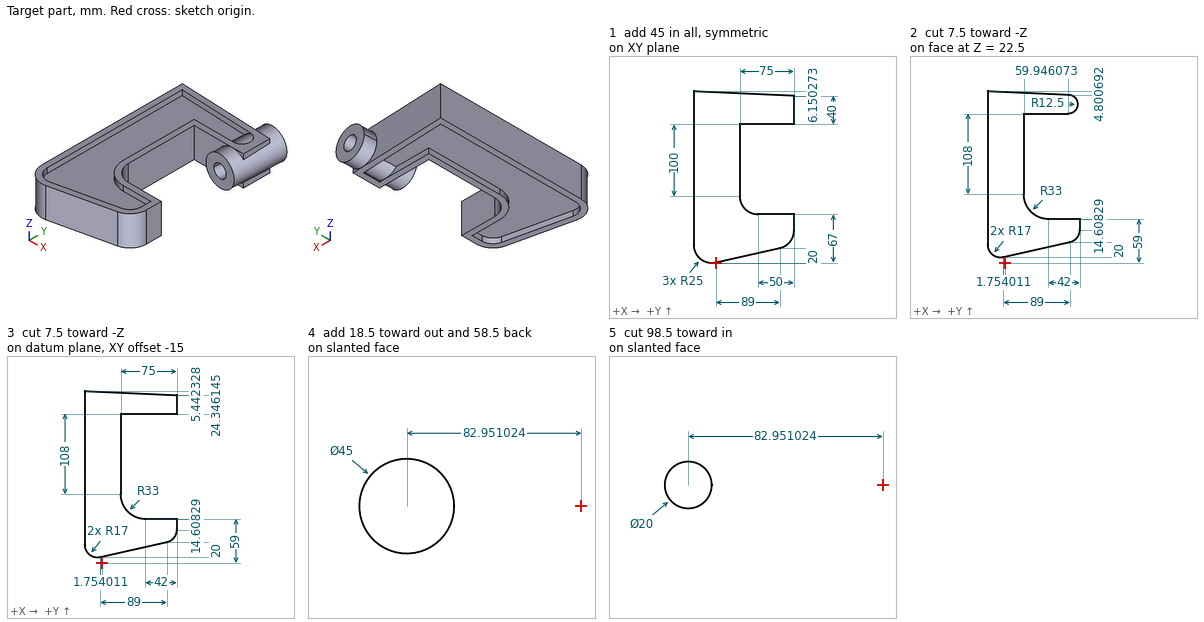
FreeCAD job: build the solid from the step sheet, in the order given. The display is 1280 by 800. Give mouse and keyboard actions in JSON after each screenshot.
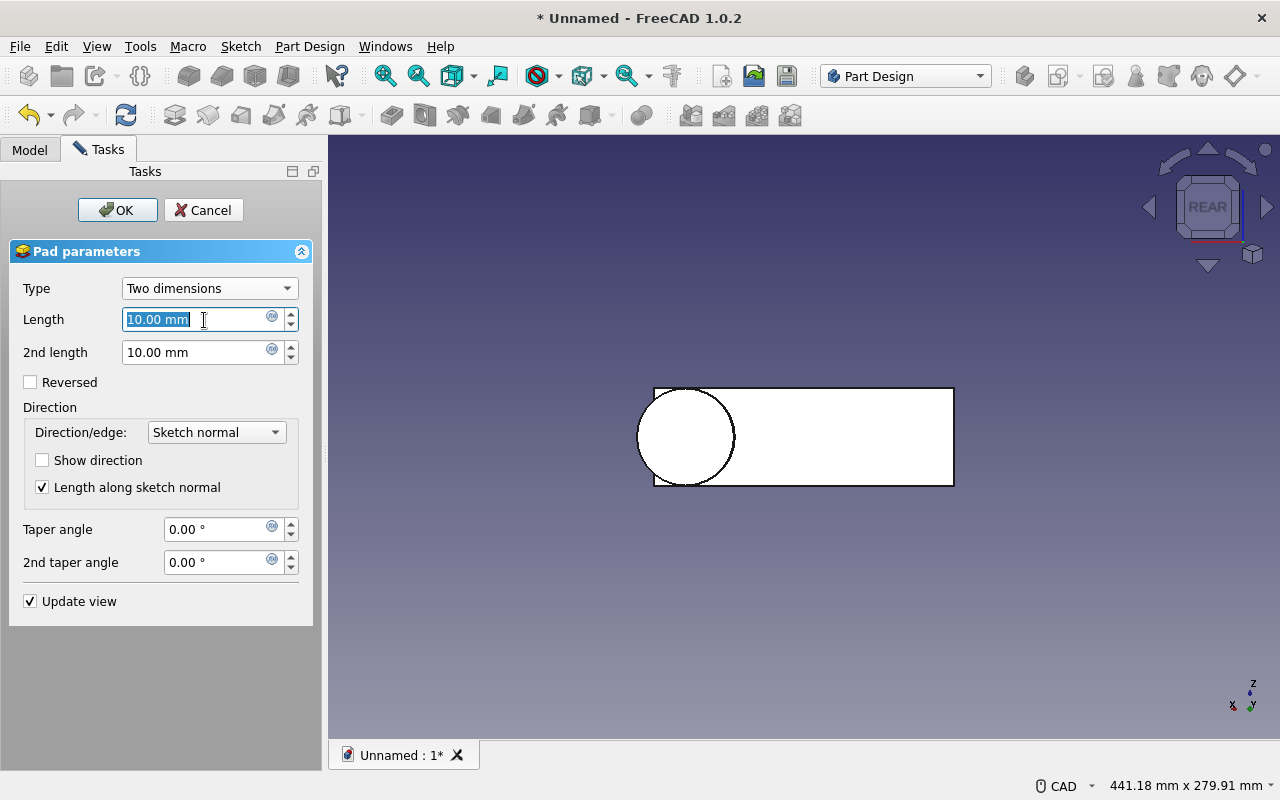
{"action": "type", "text": "18.5"}
{"action": "key", "text": "Tab"}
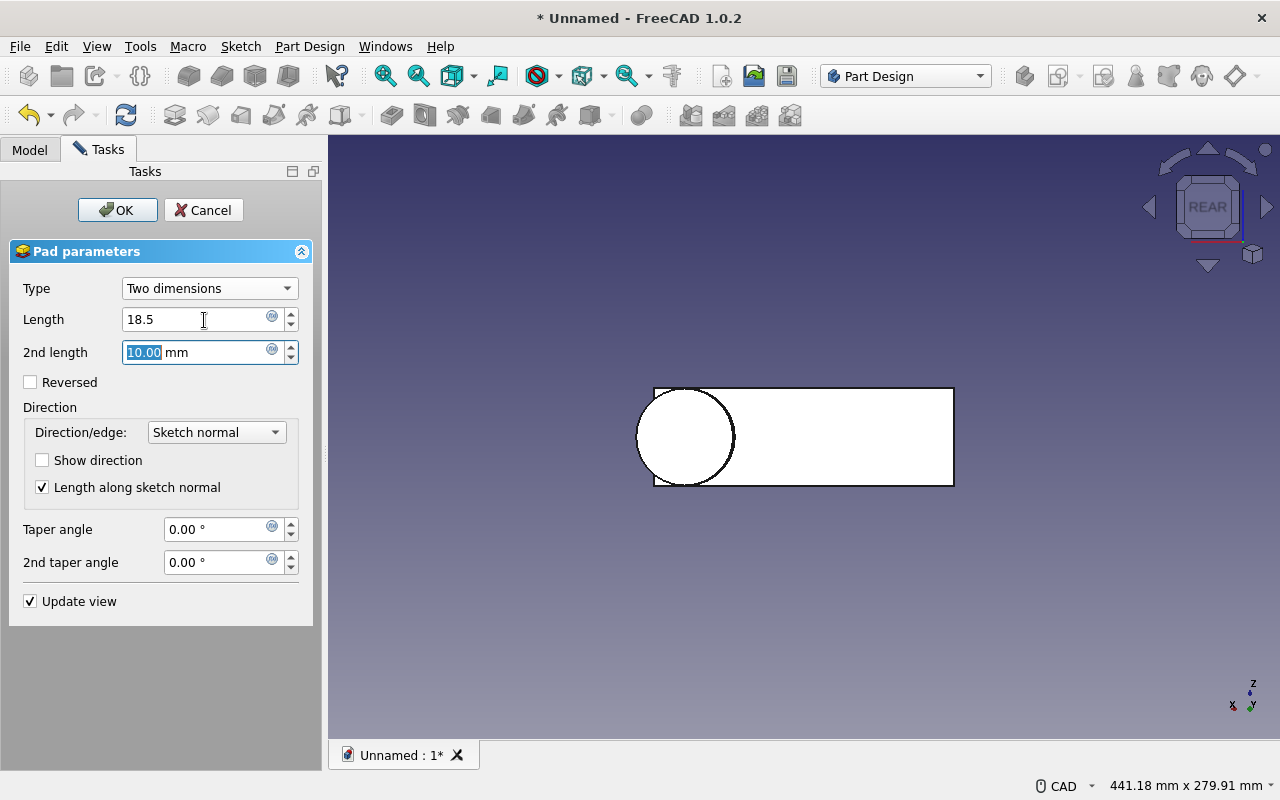
{"action": "type", "text": "58.5"}
{"action": "key", "text": "Tab"}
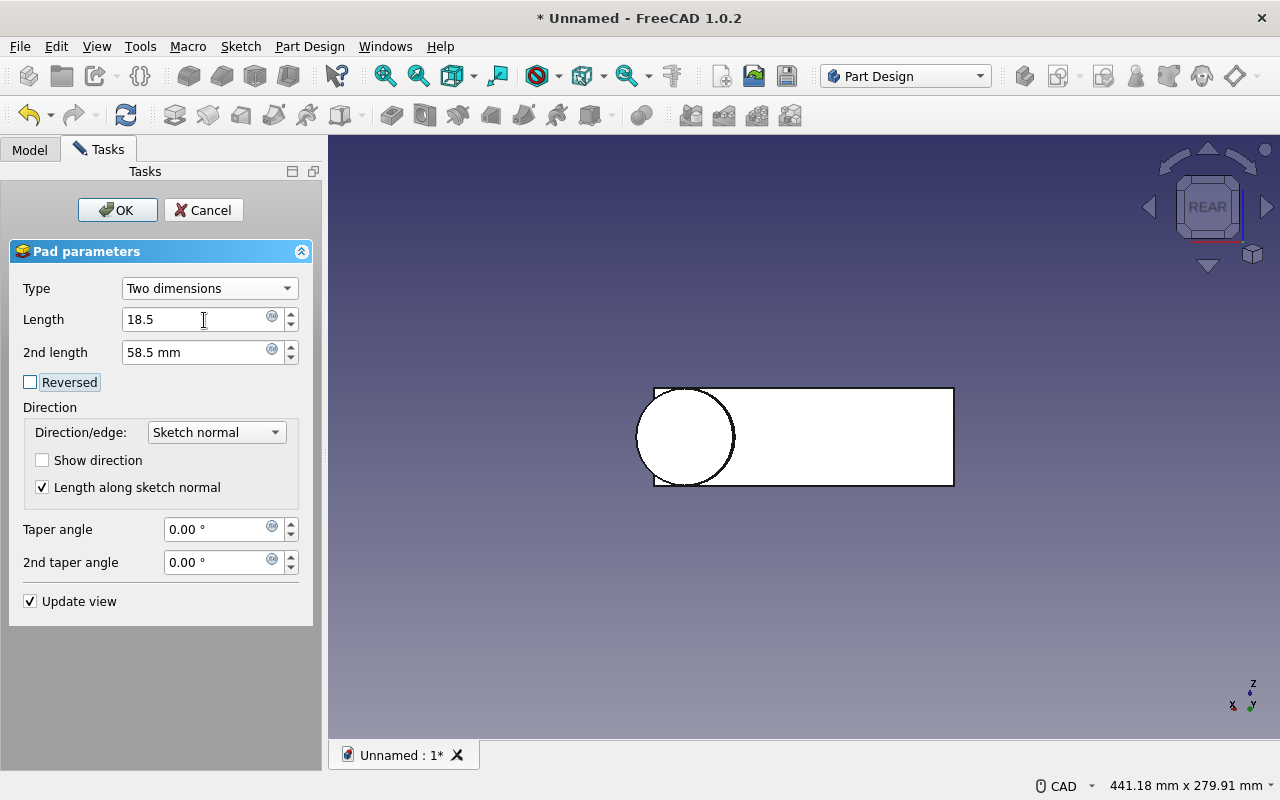
{"action": "left_click", "coordinate": [118, 210]}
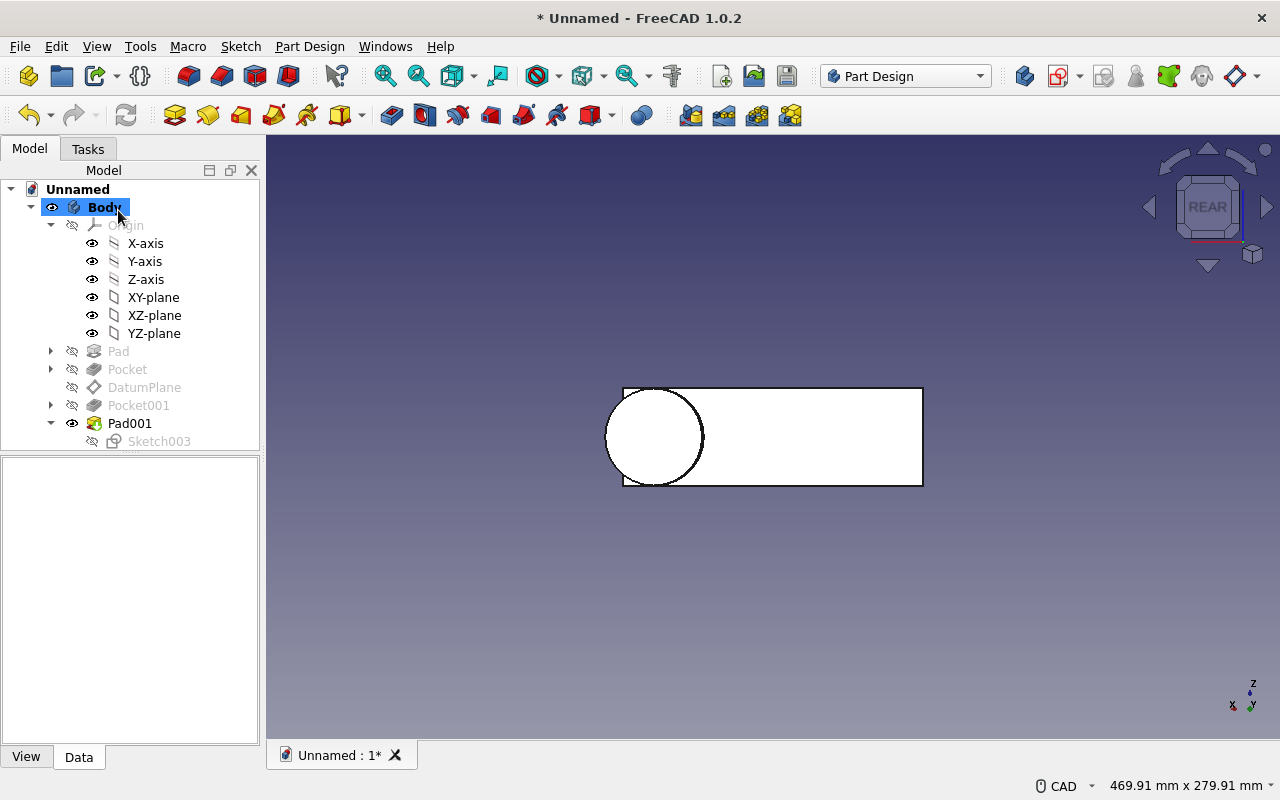
{"action": "left_click", "coordinate": [386, 76]}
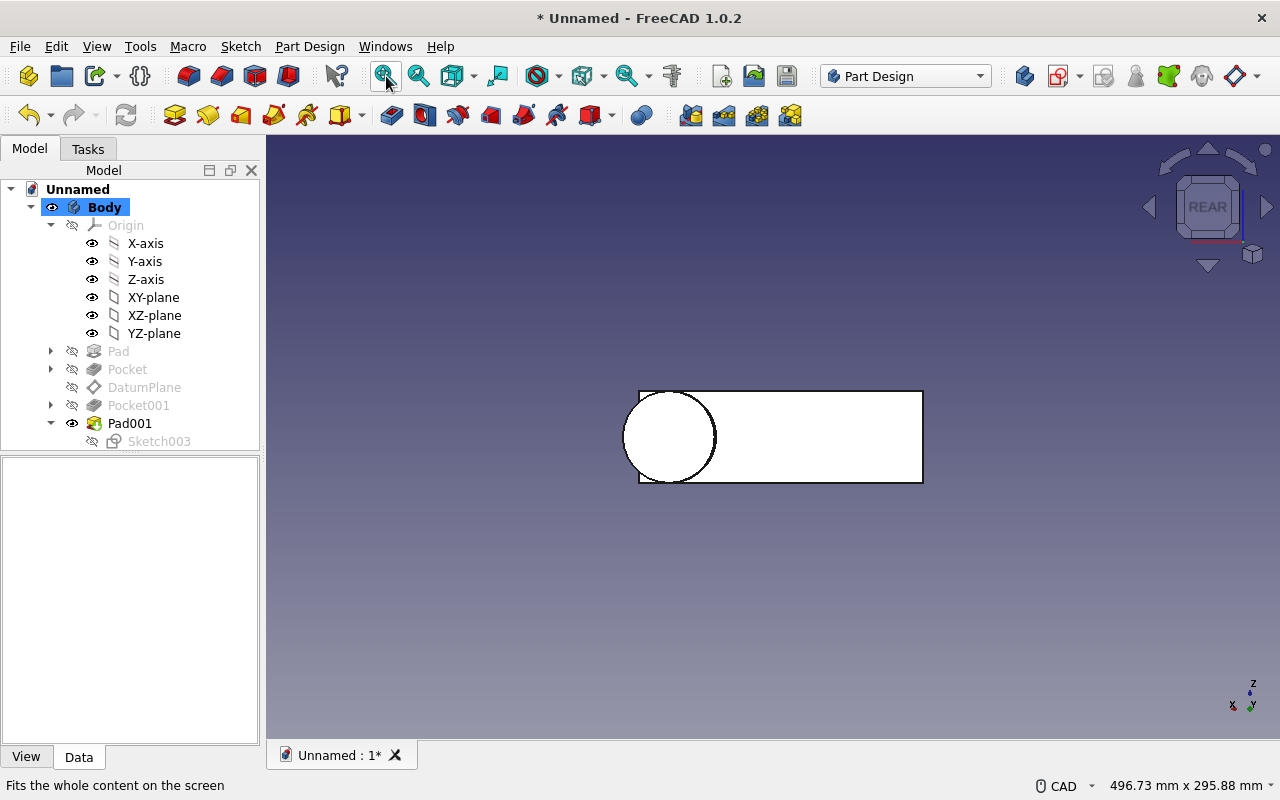
{"action": "left_click", "coordinate": [669, 436]}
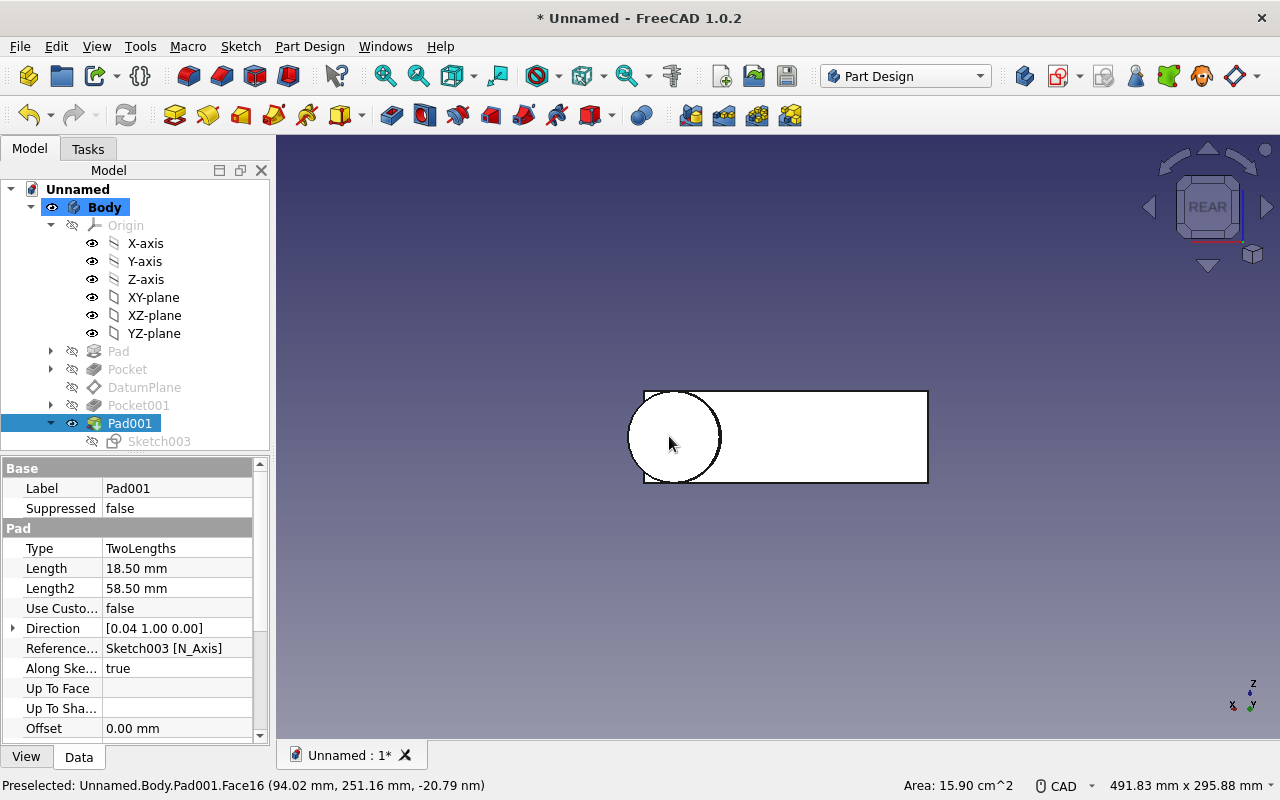
{"action": "left_click", "coordinate": [1058, 76]}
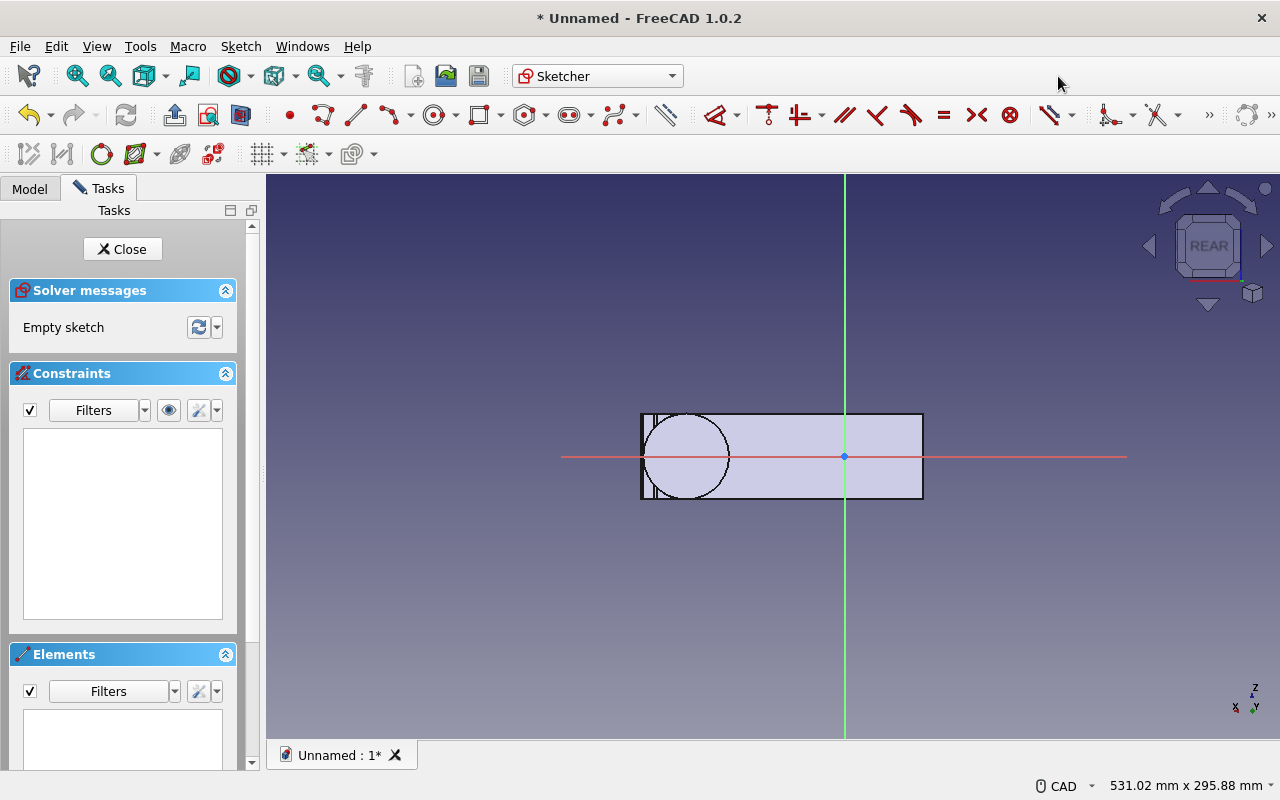
{"action": "scroll", "coordinate": [684, 457], "scroll_direction": "up", "scroll_amount": 11}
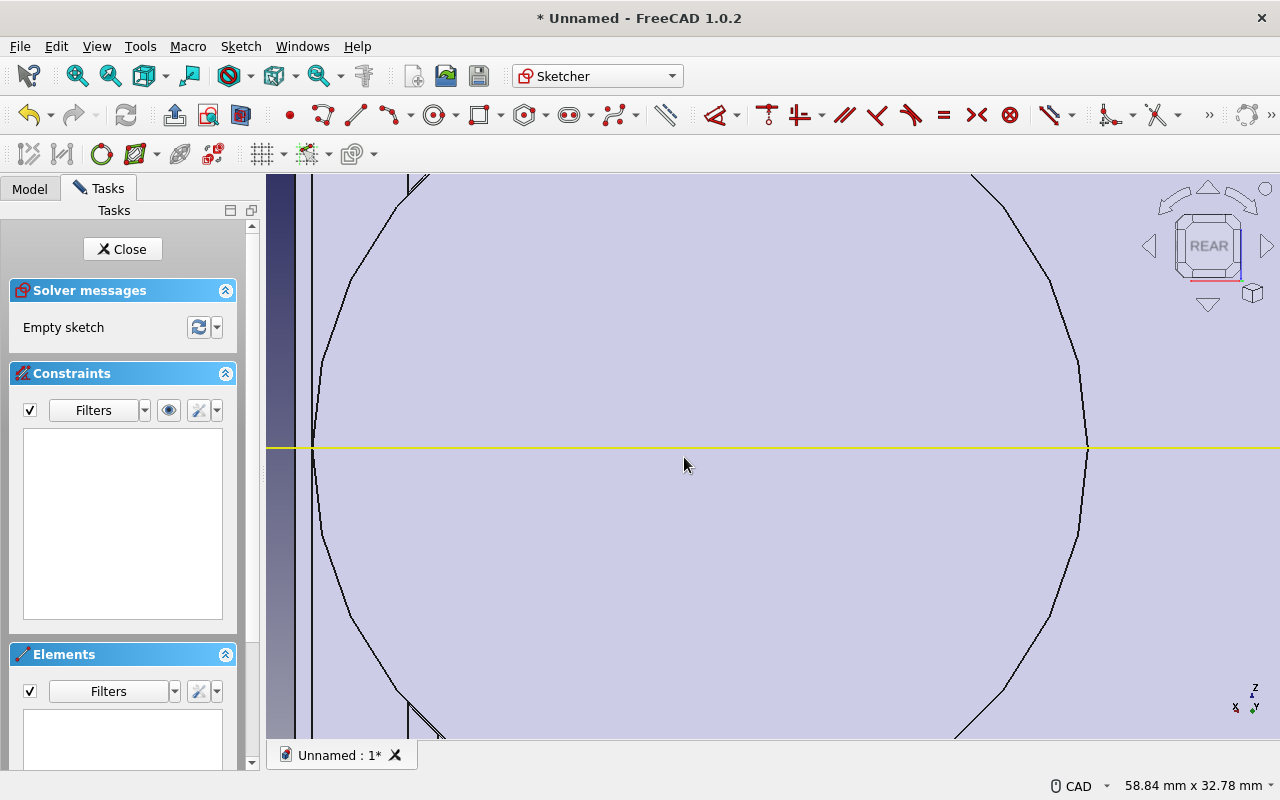
{"action": "left_click", "coordinate": [434, 116]}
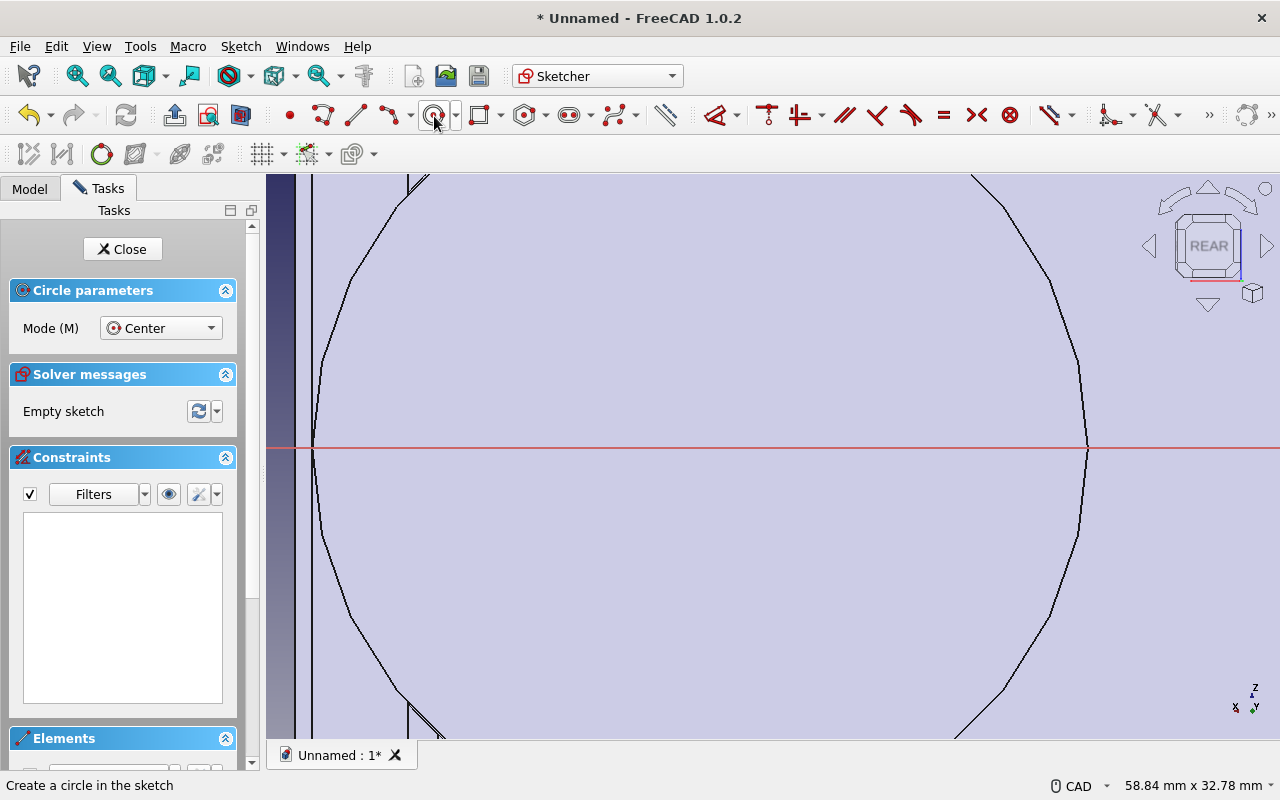
{"action": "left_click", "coordinate": [700, 448]}
{"action": "left_click", "coordinate": [822, 327]}
{"action": "key", "text": "Escape"}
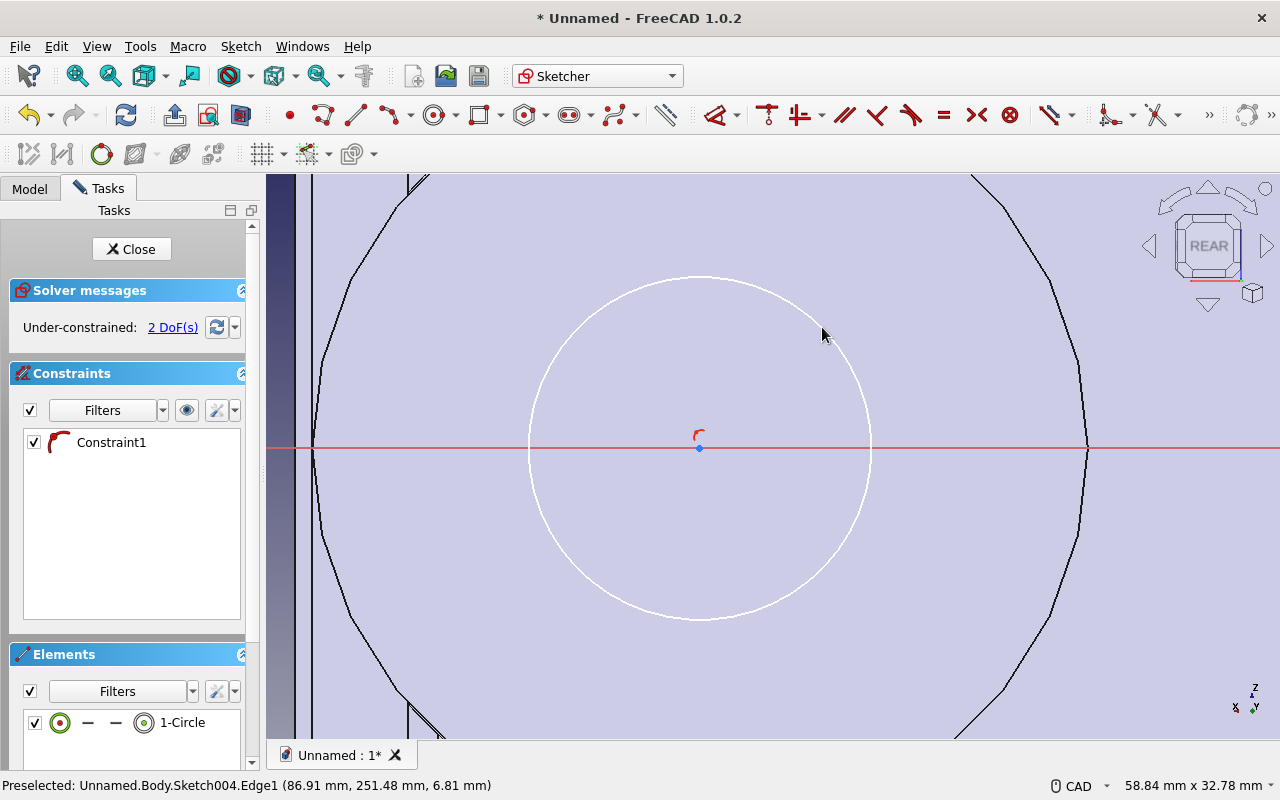
{"action": "left_click", "coordinate": [714, 116]}